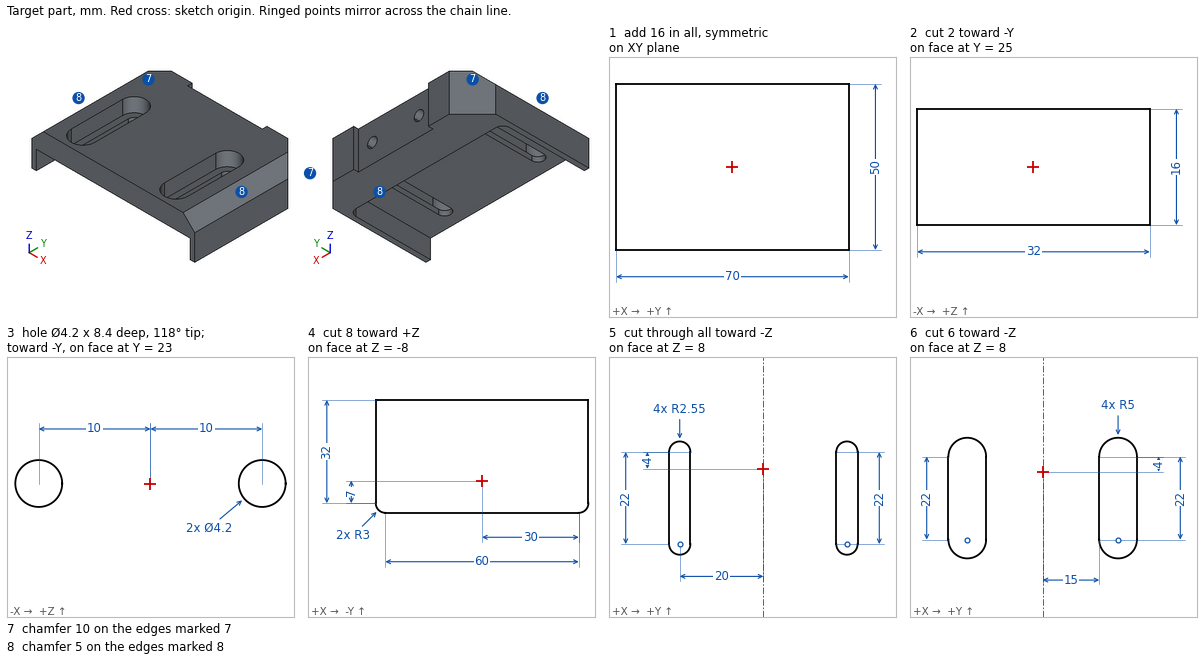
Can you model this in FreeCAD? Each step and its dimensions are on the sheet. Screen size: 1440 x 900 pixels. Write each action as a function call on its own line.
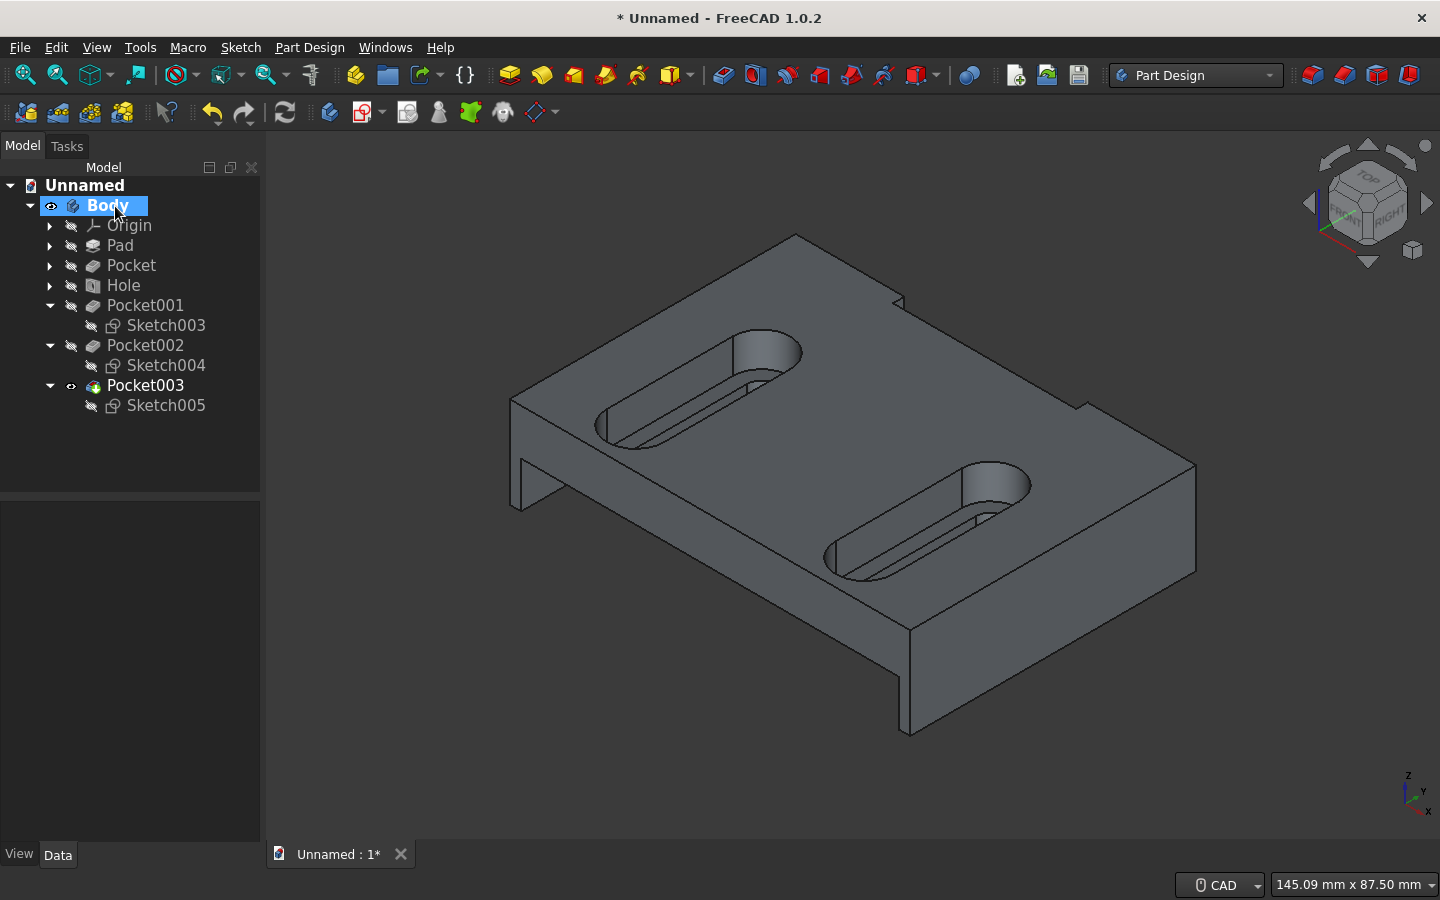
key(1)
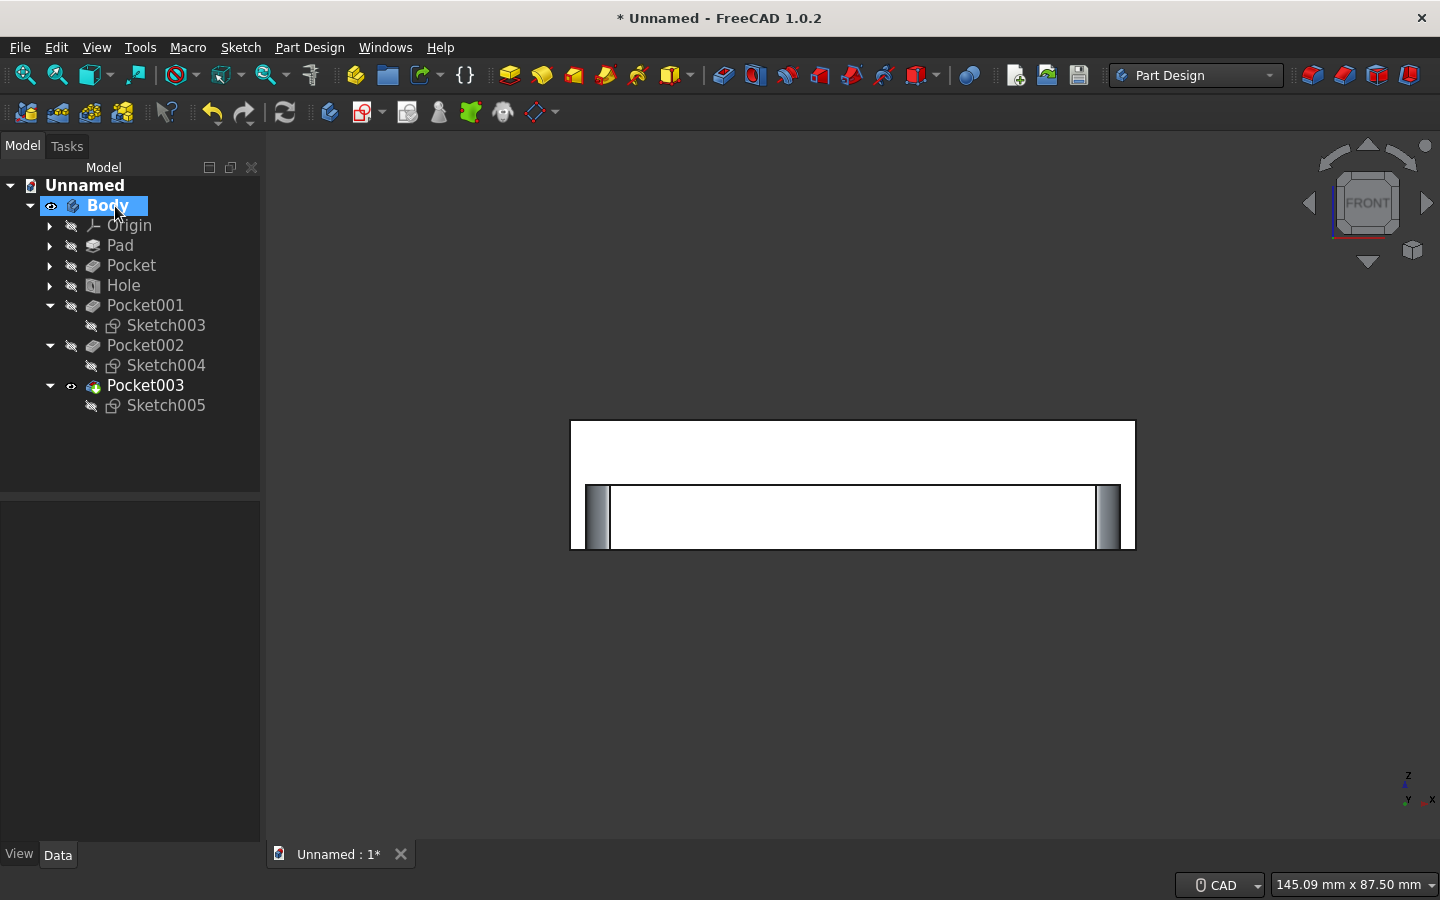
key(3)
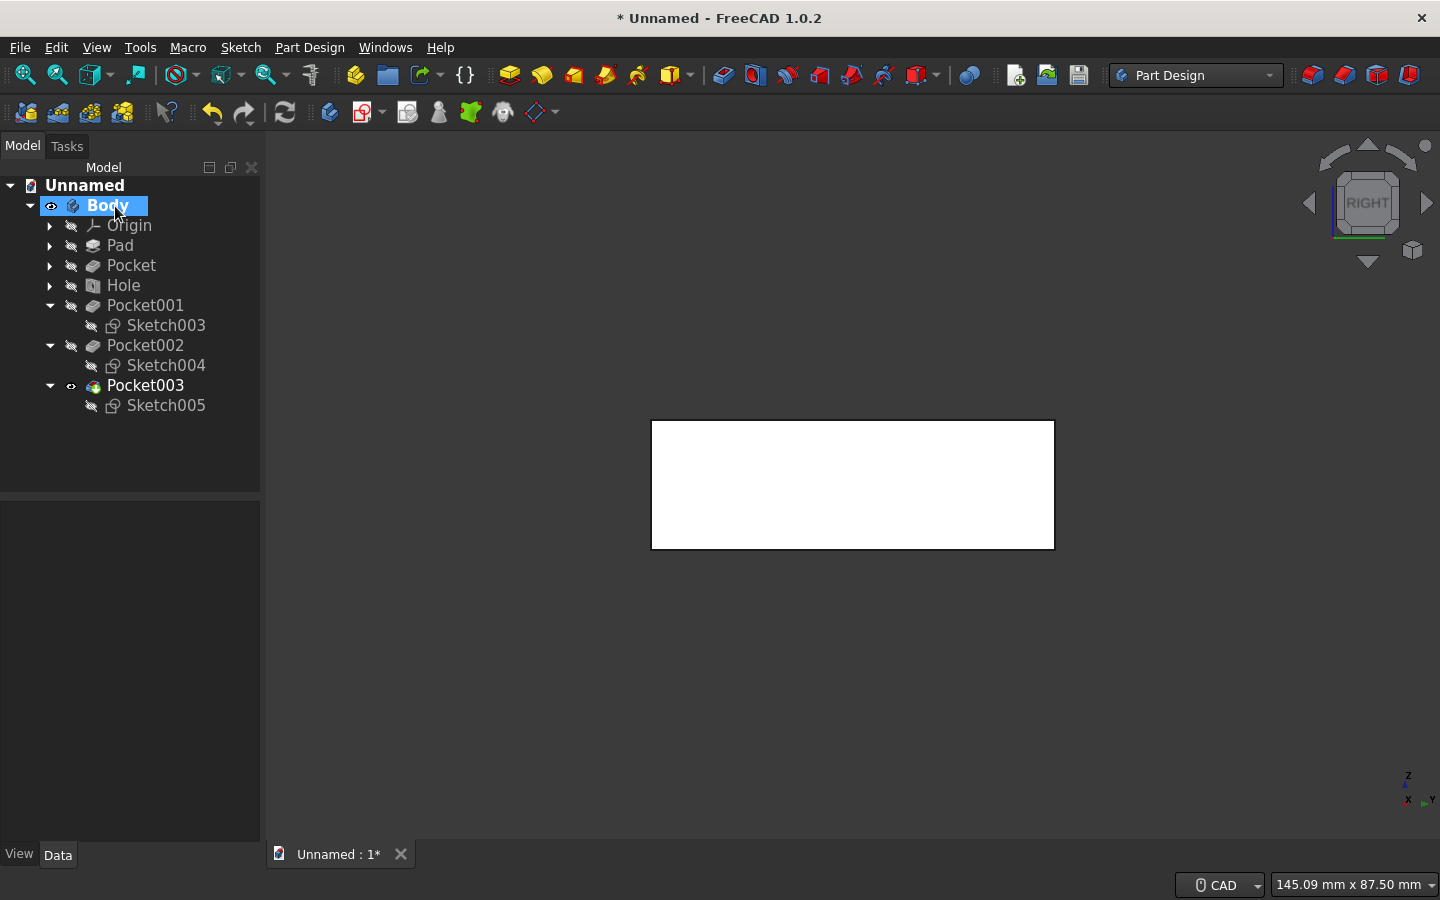
click(26, 76)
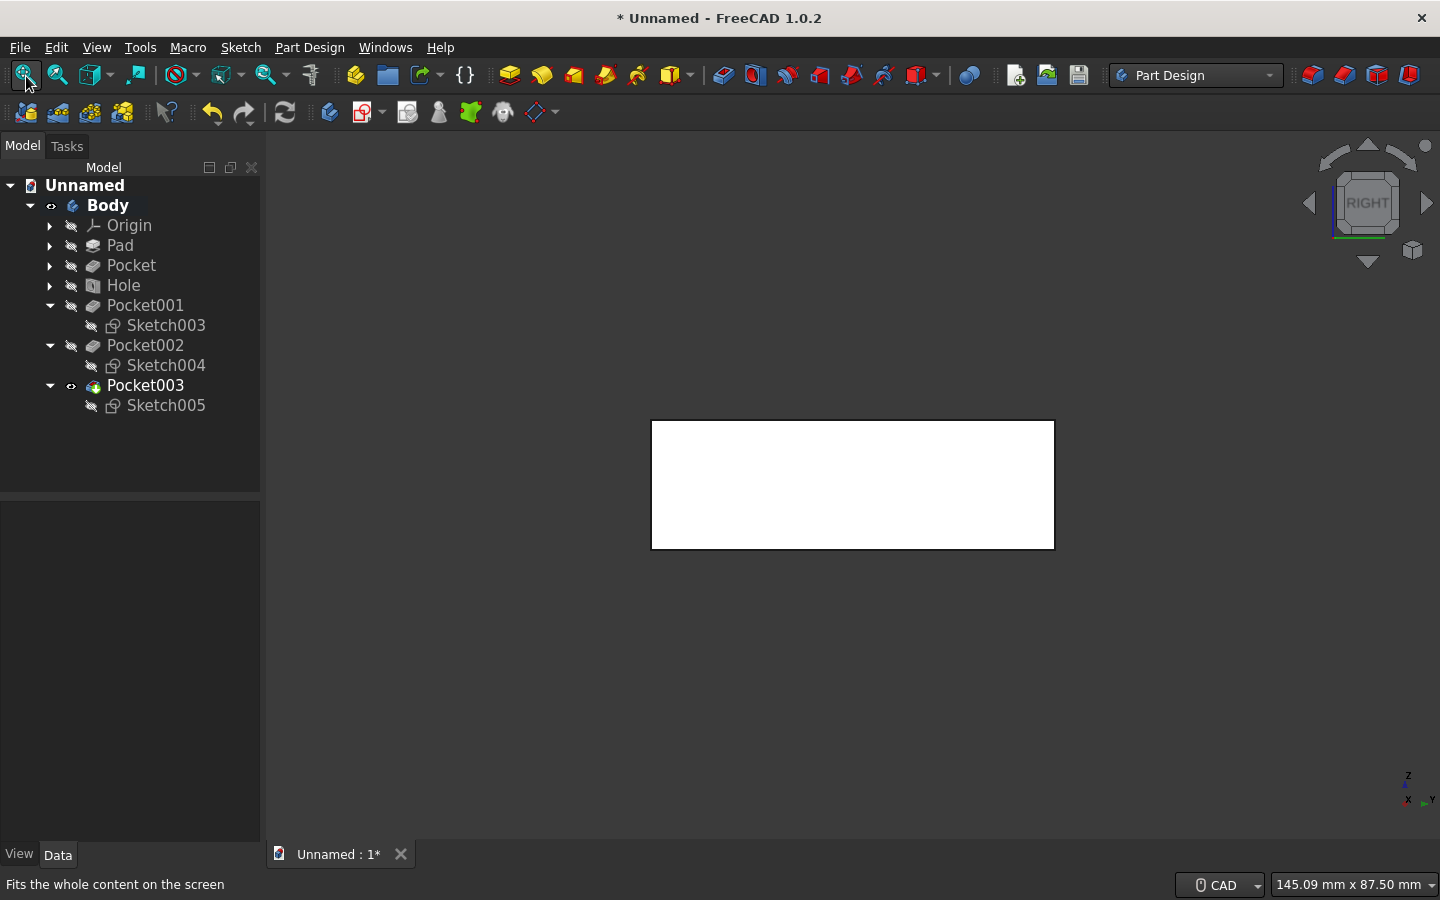
click(1055, 484)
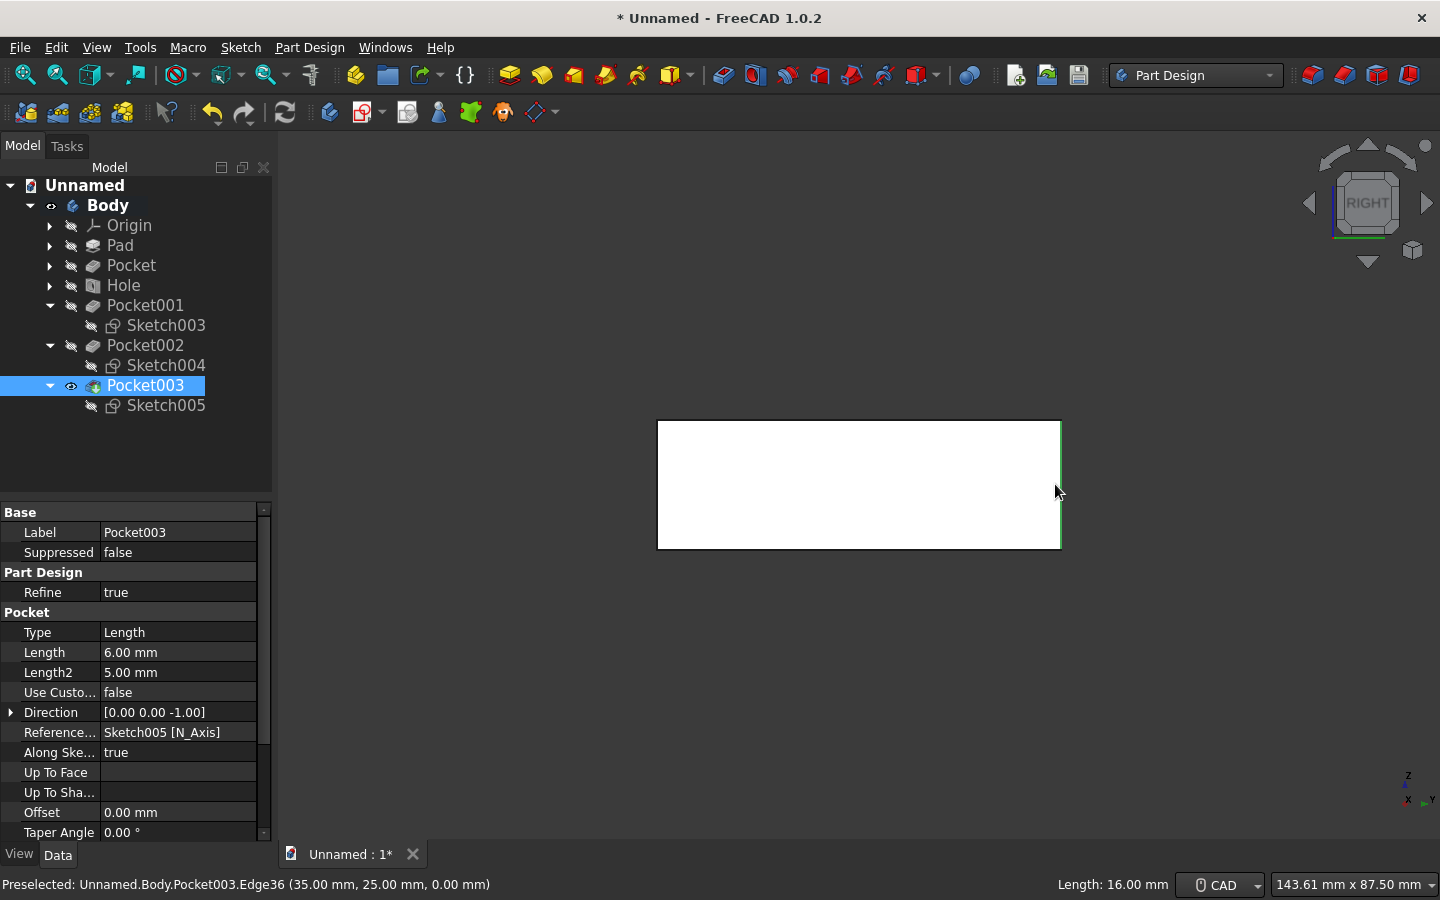
key(5)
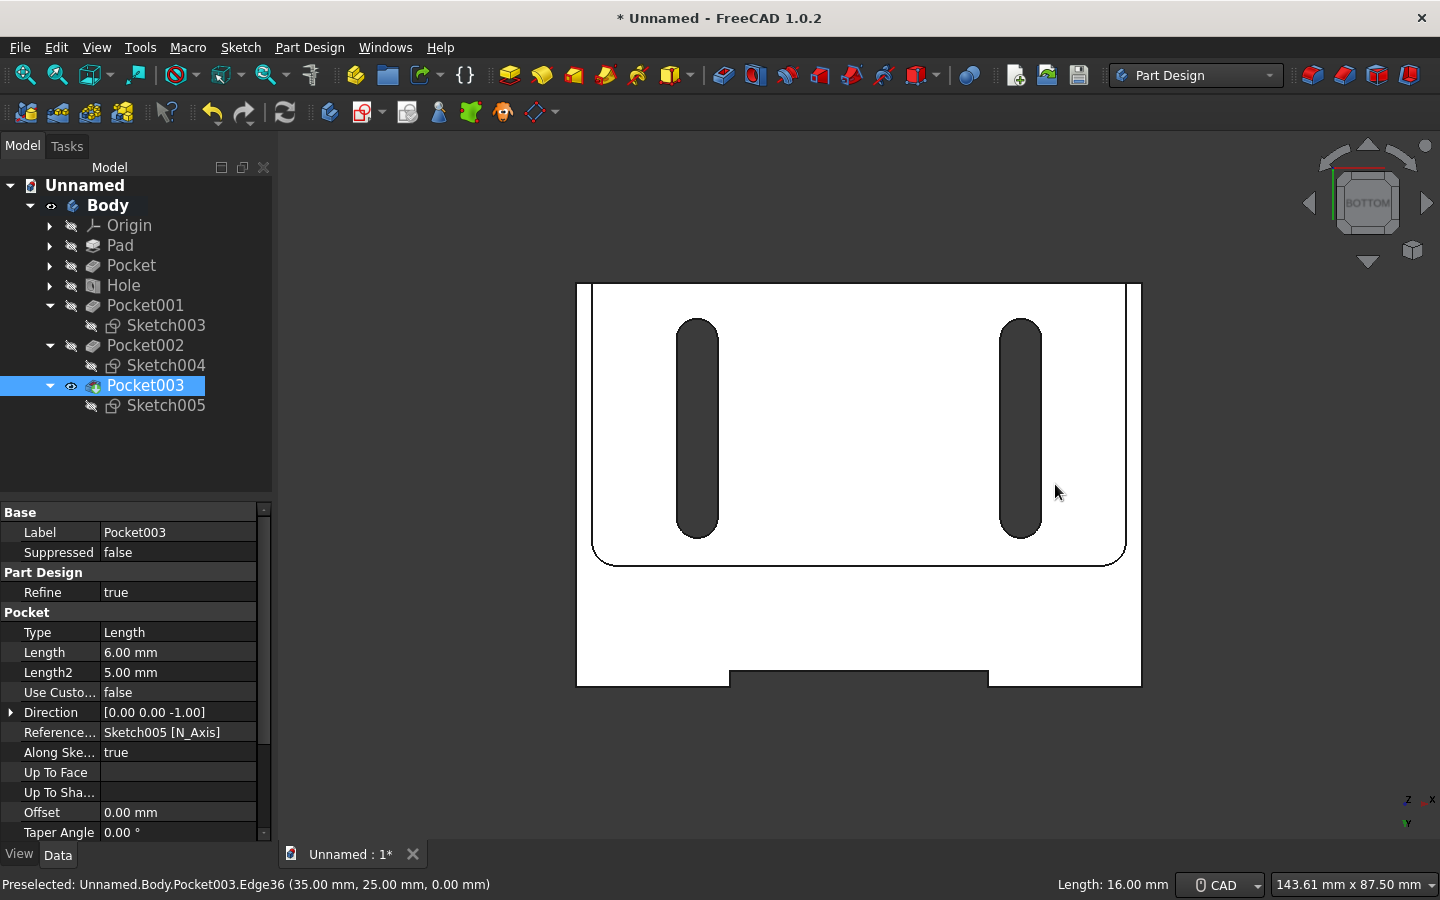
key(4)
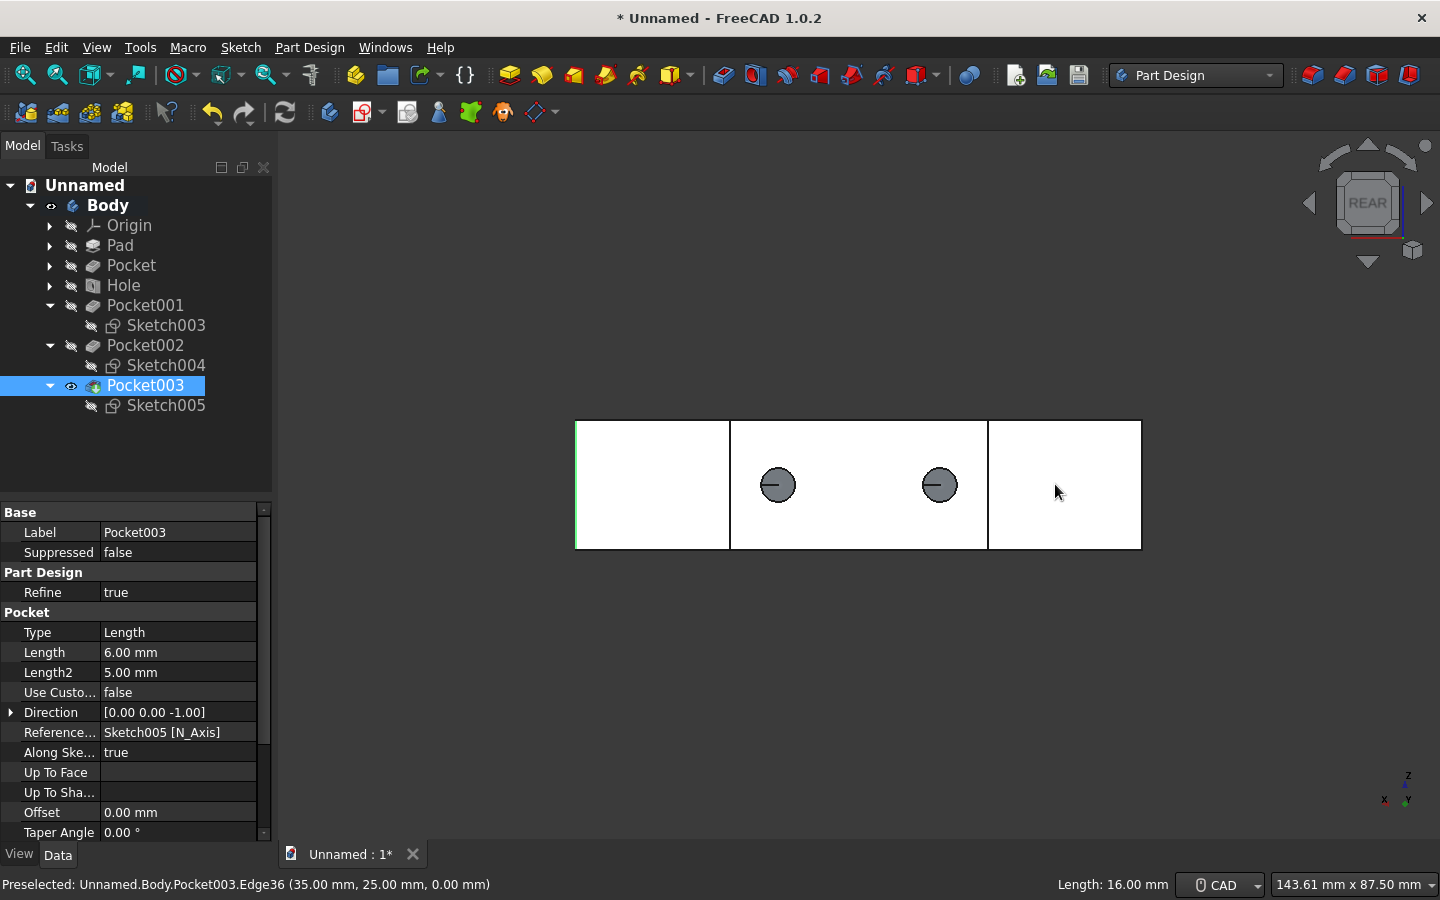
click(1142, 484, ctrl)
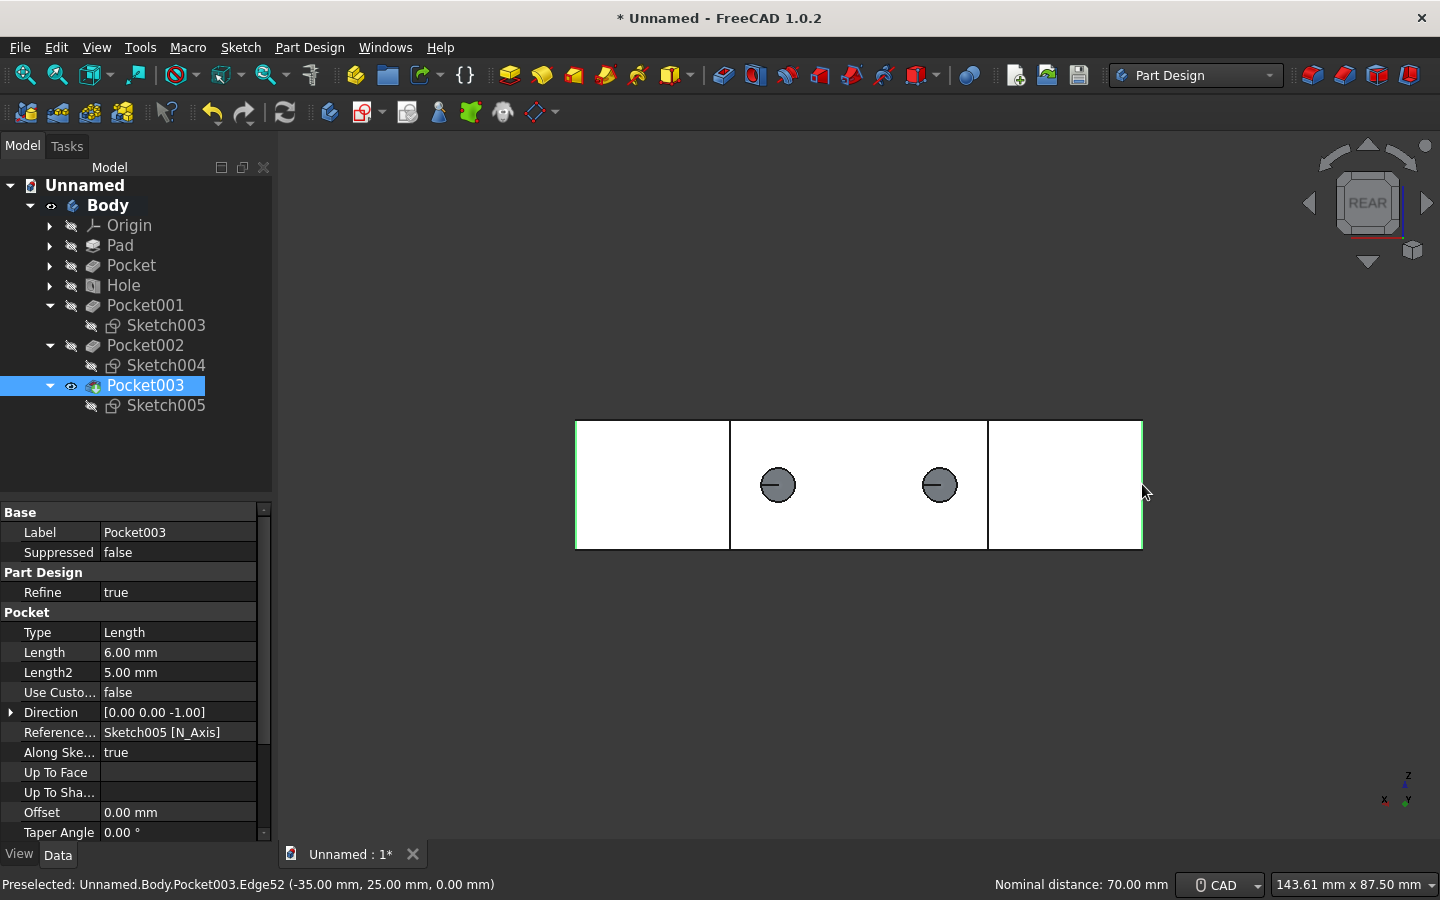
click(1346, 76)